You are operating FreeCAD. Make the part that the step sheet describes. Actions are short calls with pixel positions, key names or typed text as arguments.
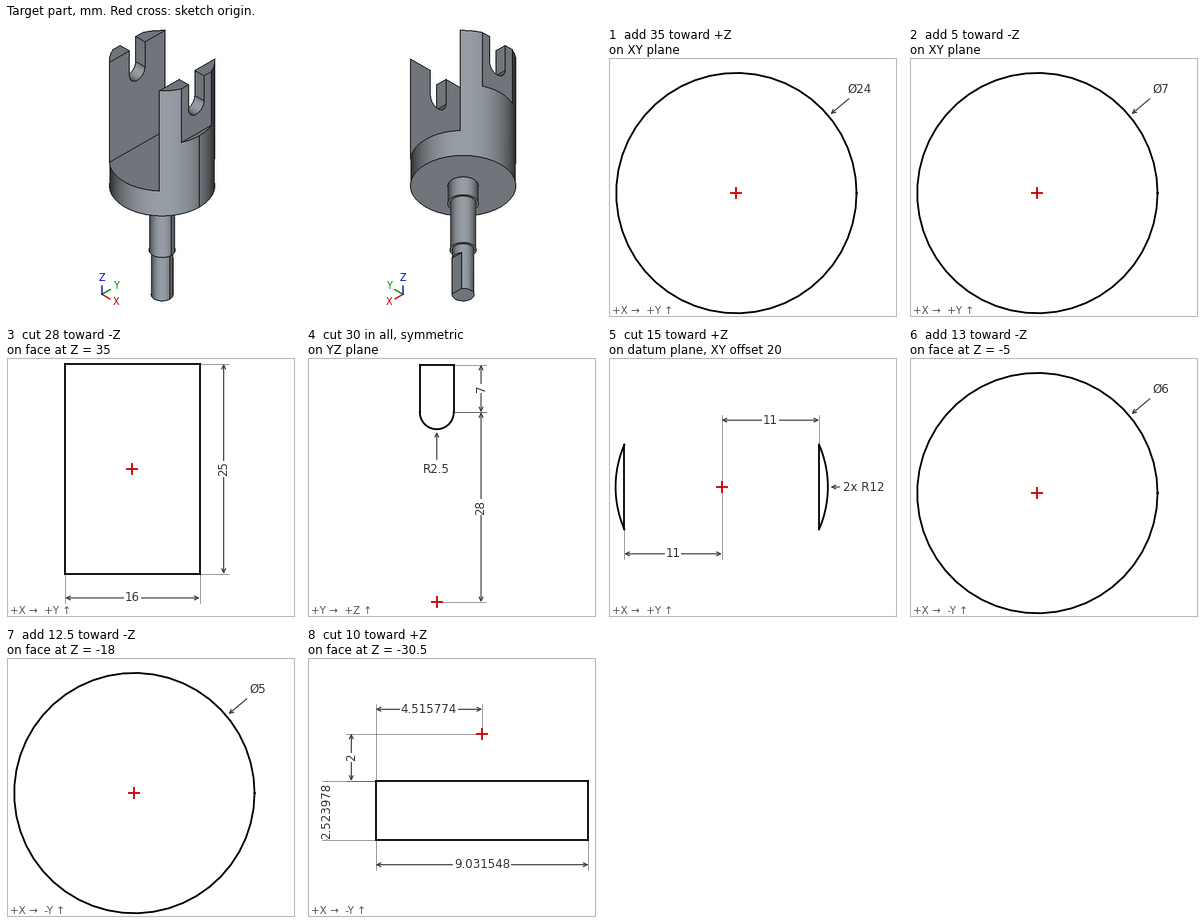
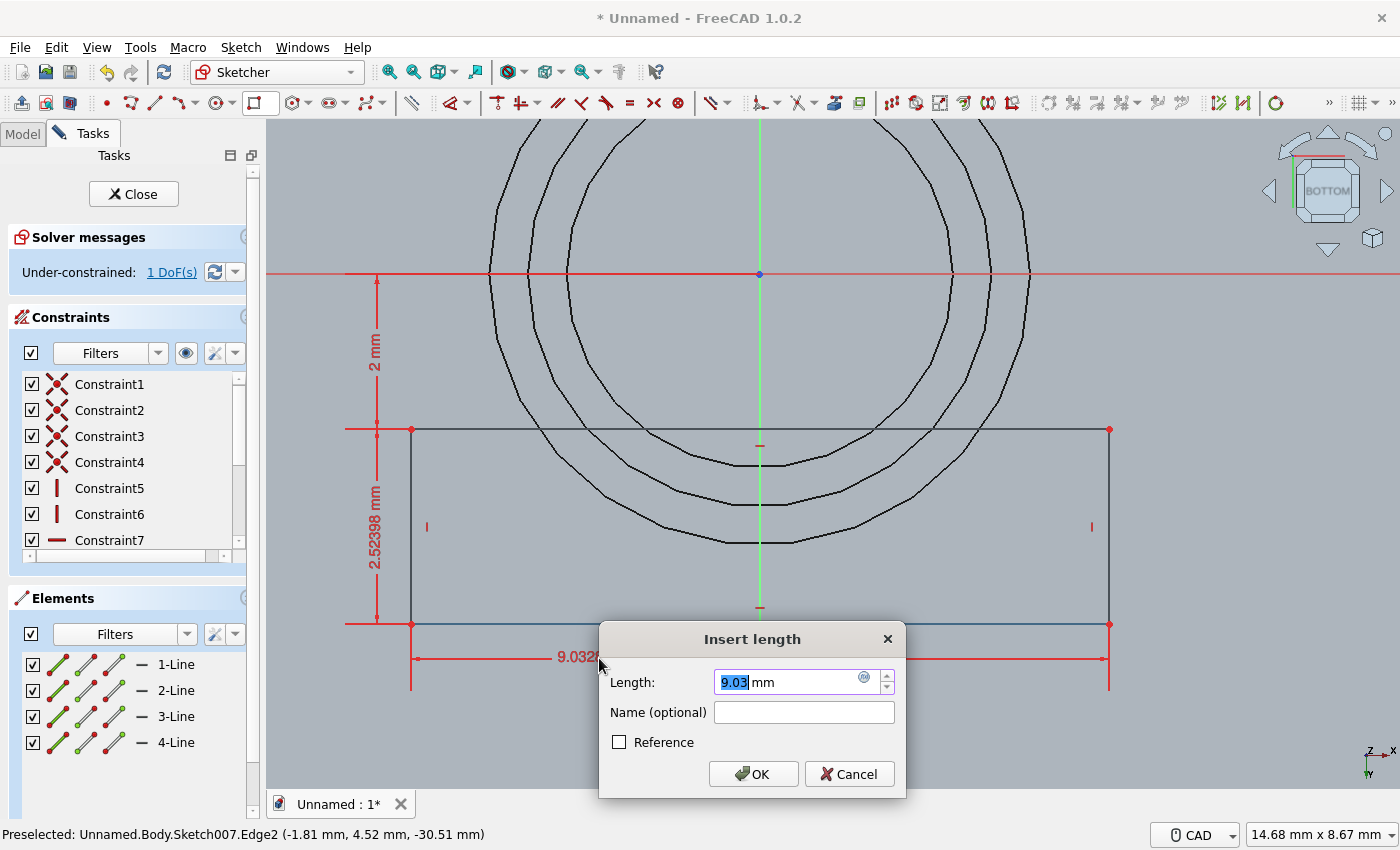
text(9.031548)
key(Return)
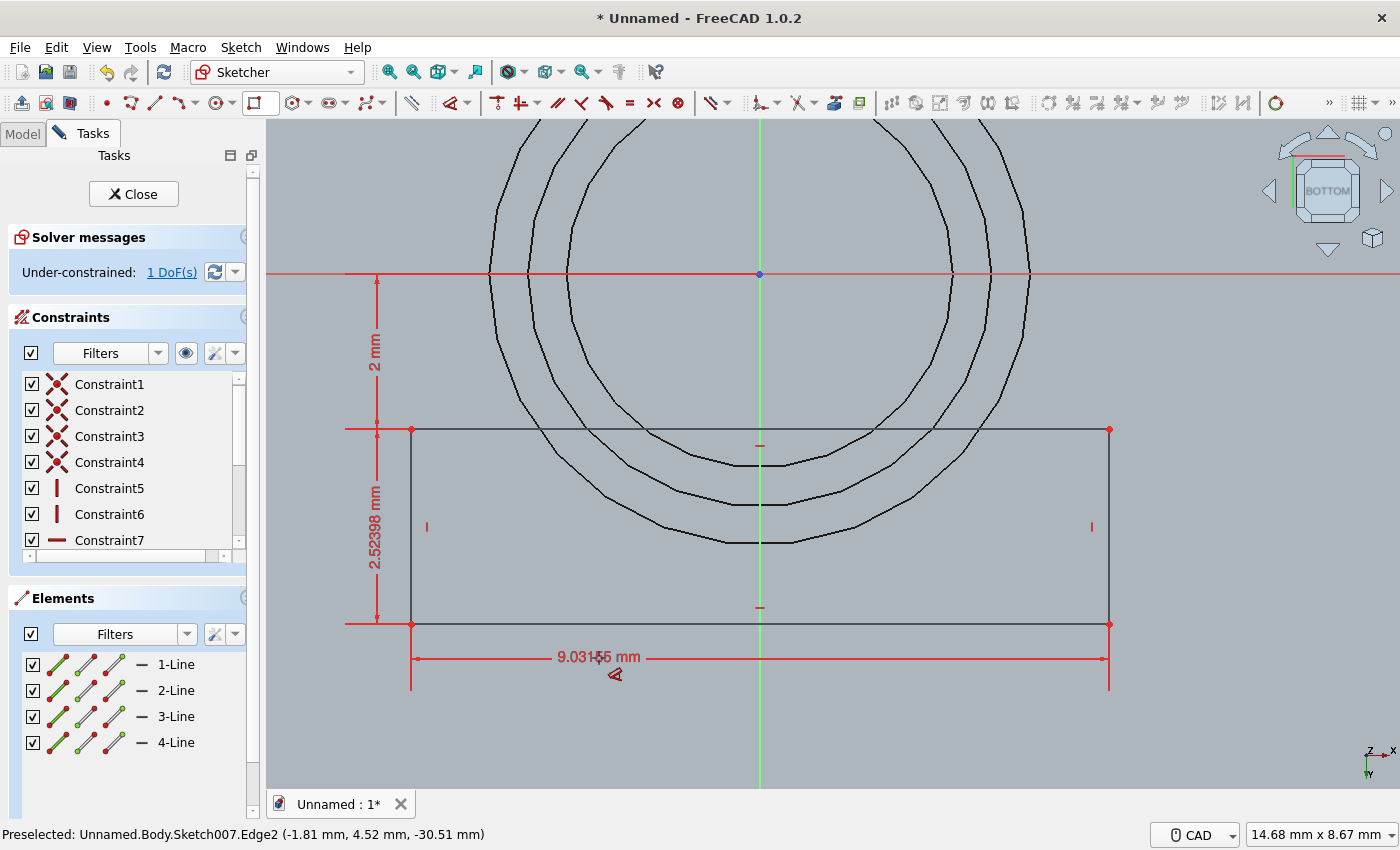
click(411, 429)
click(585, 240)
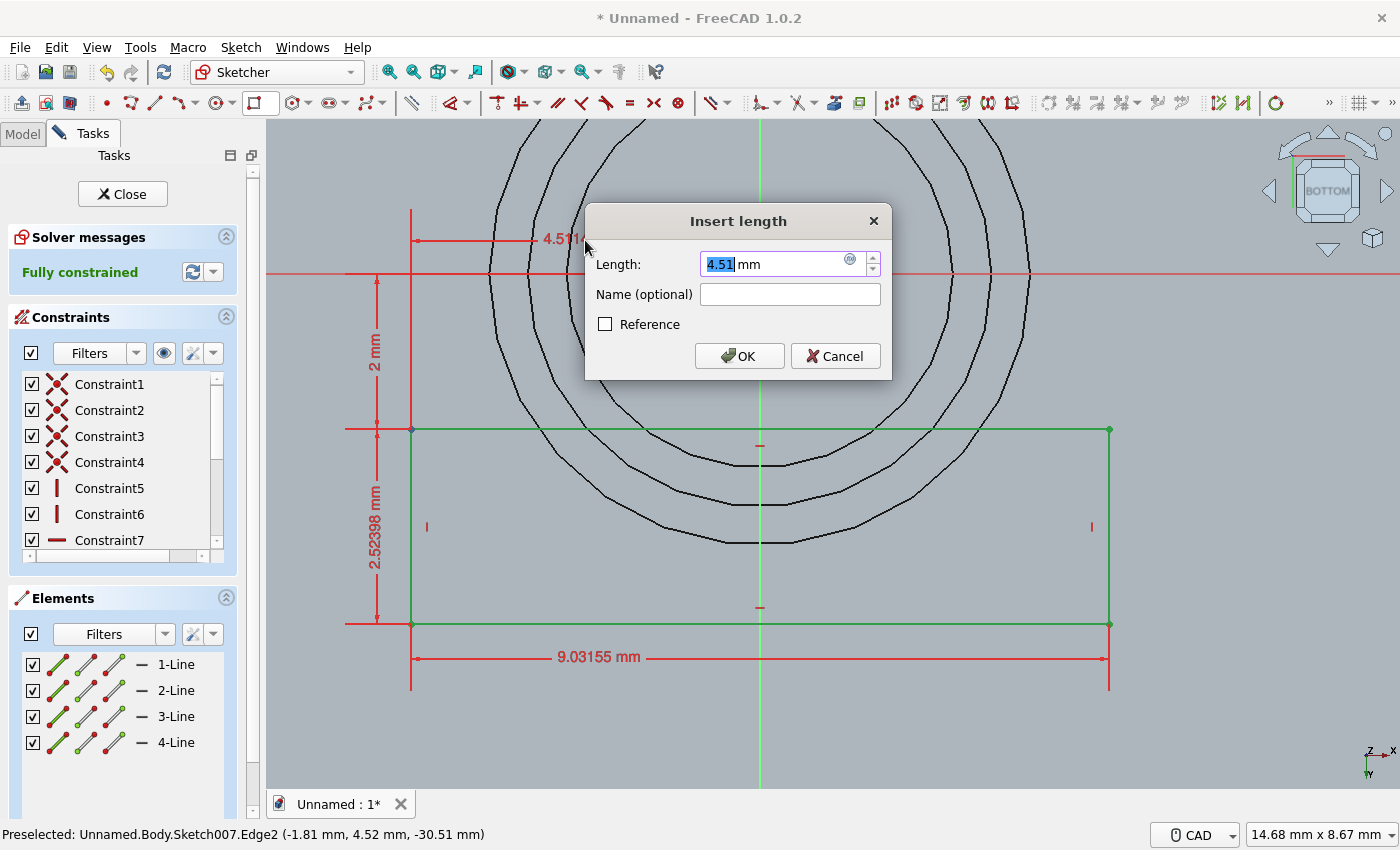
text(4.515774)
key(Return)
key(Escape)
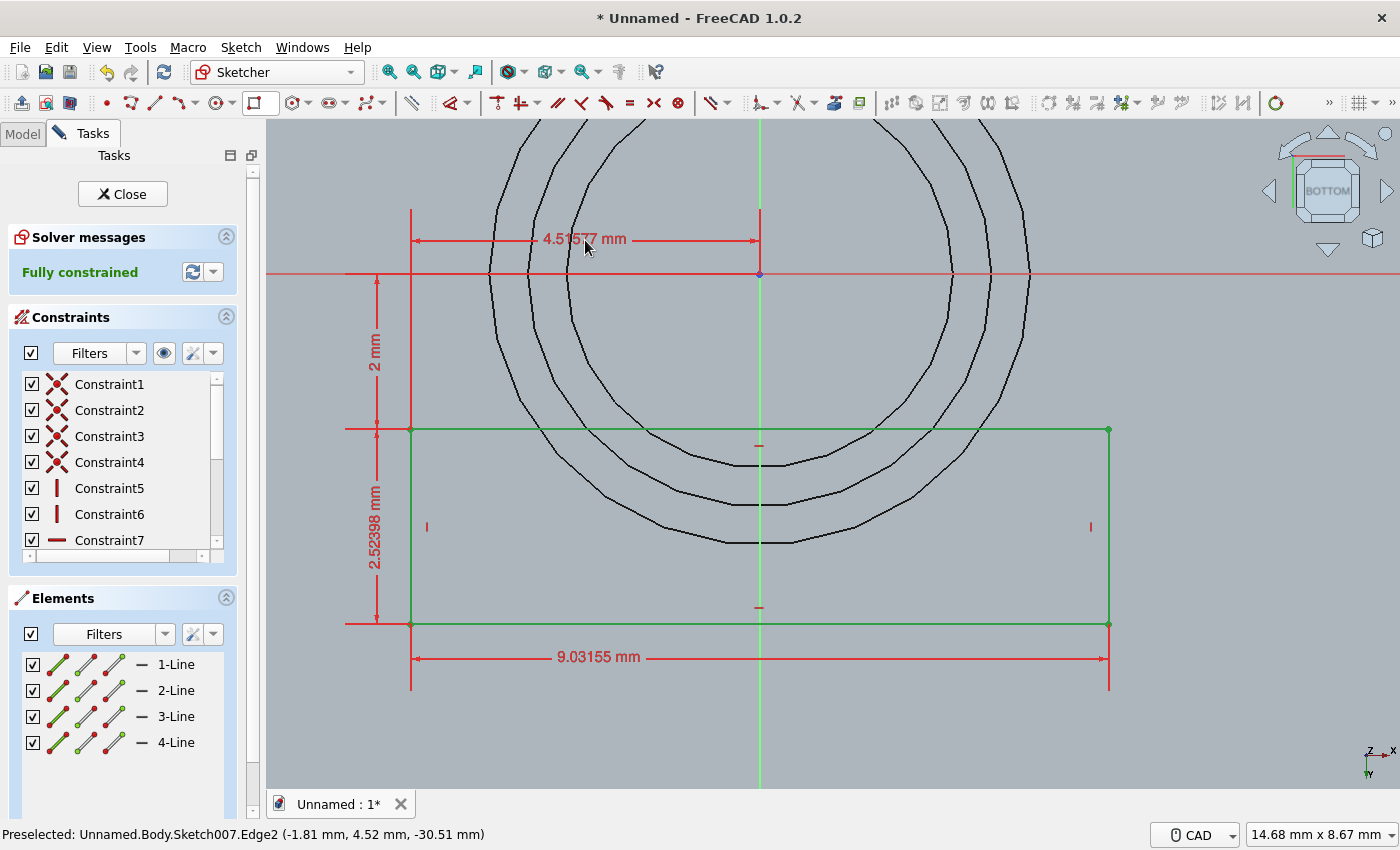
click(123, 194)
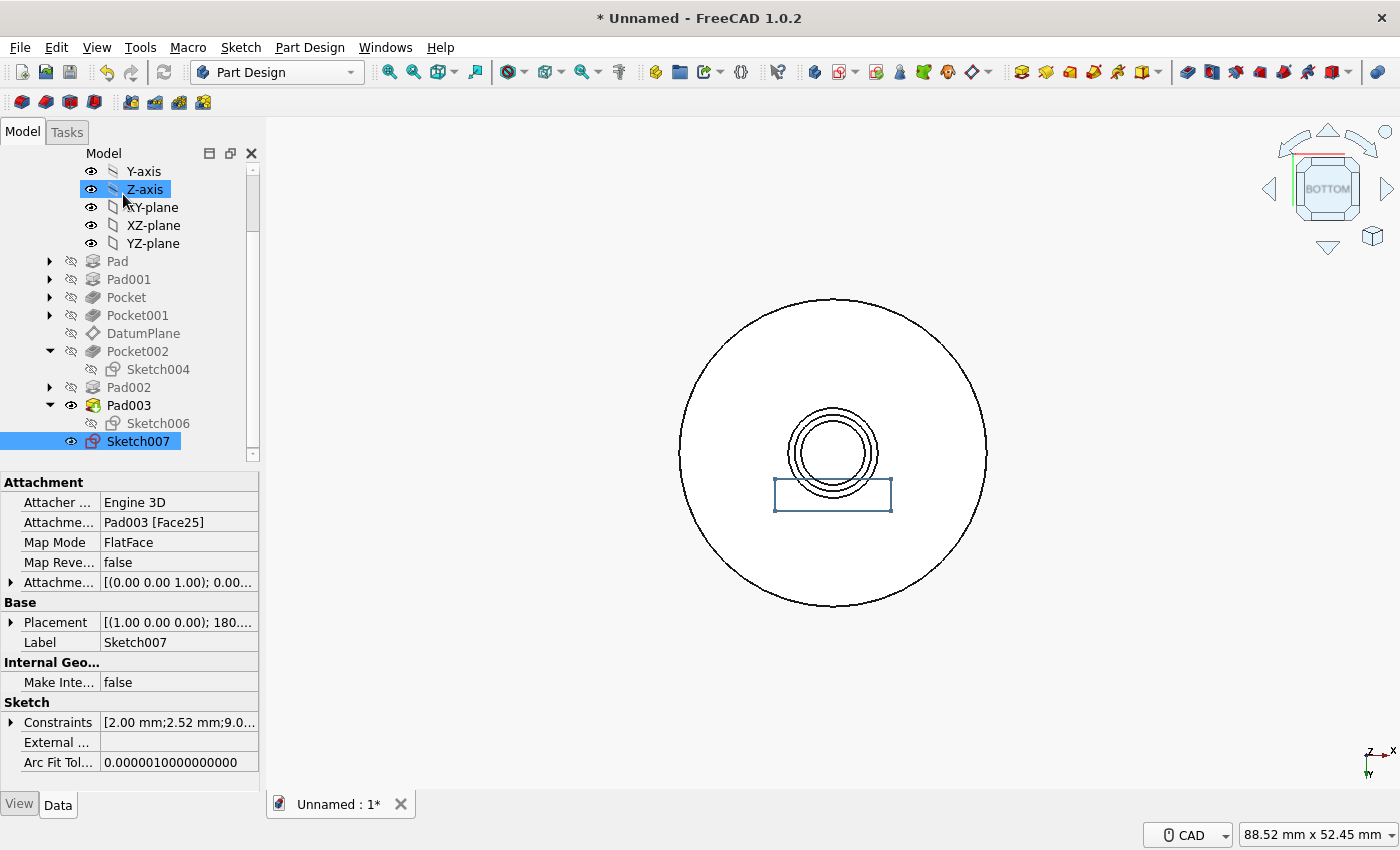
click(1188, 72)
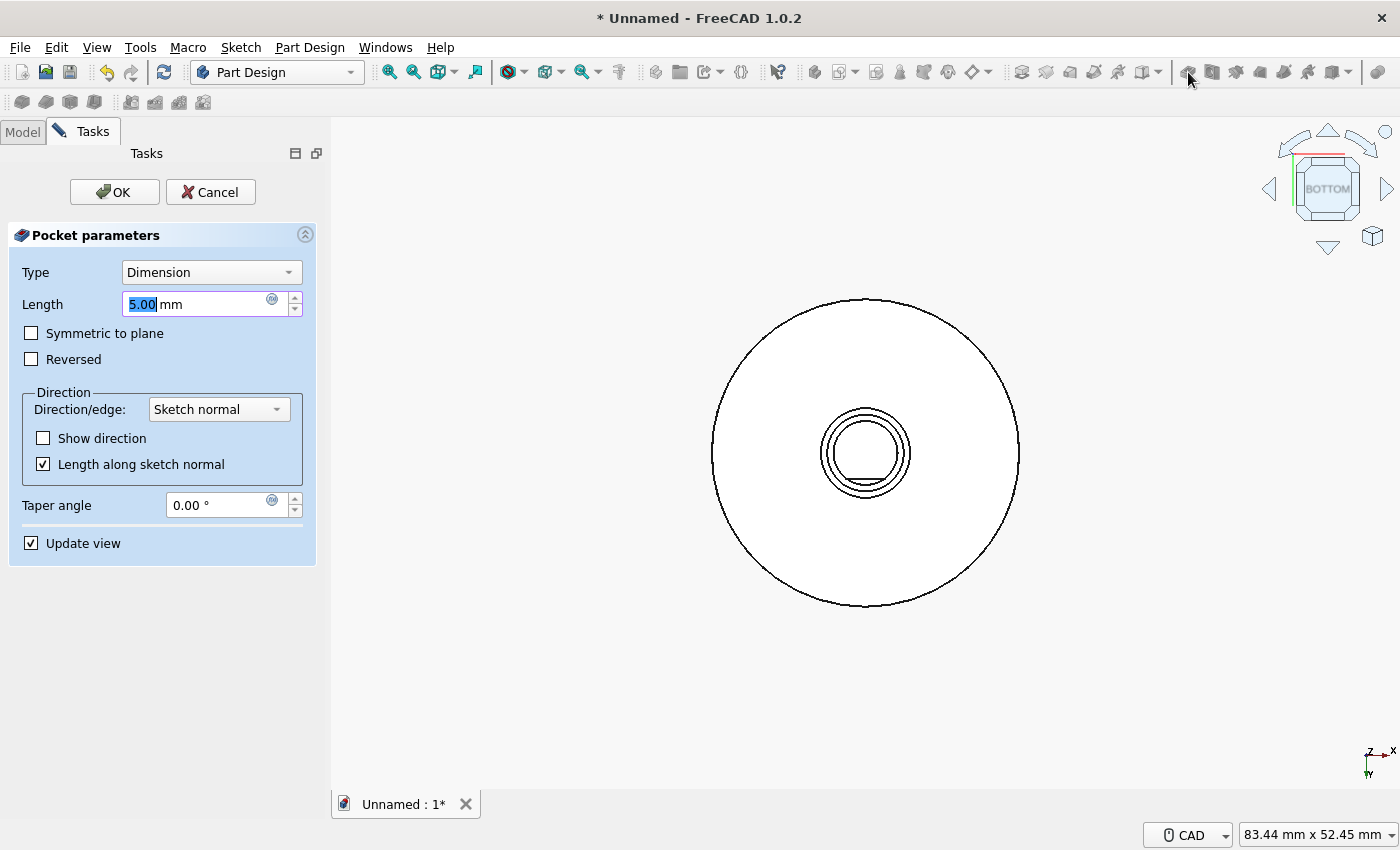
text(10)
key(Tab)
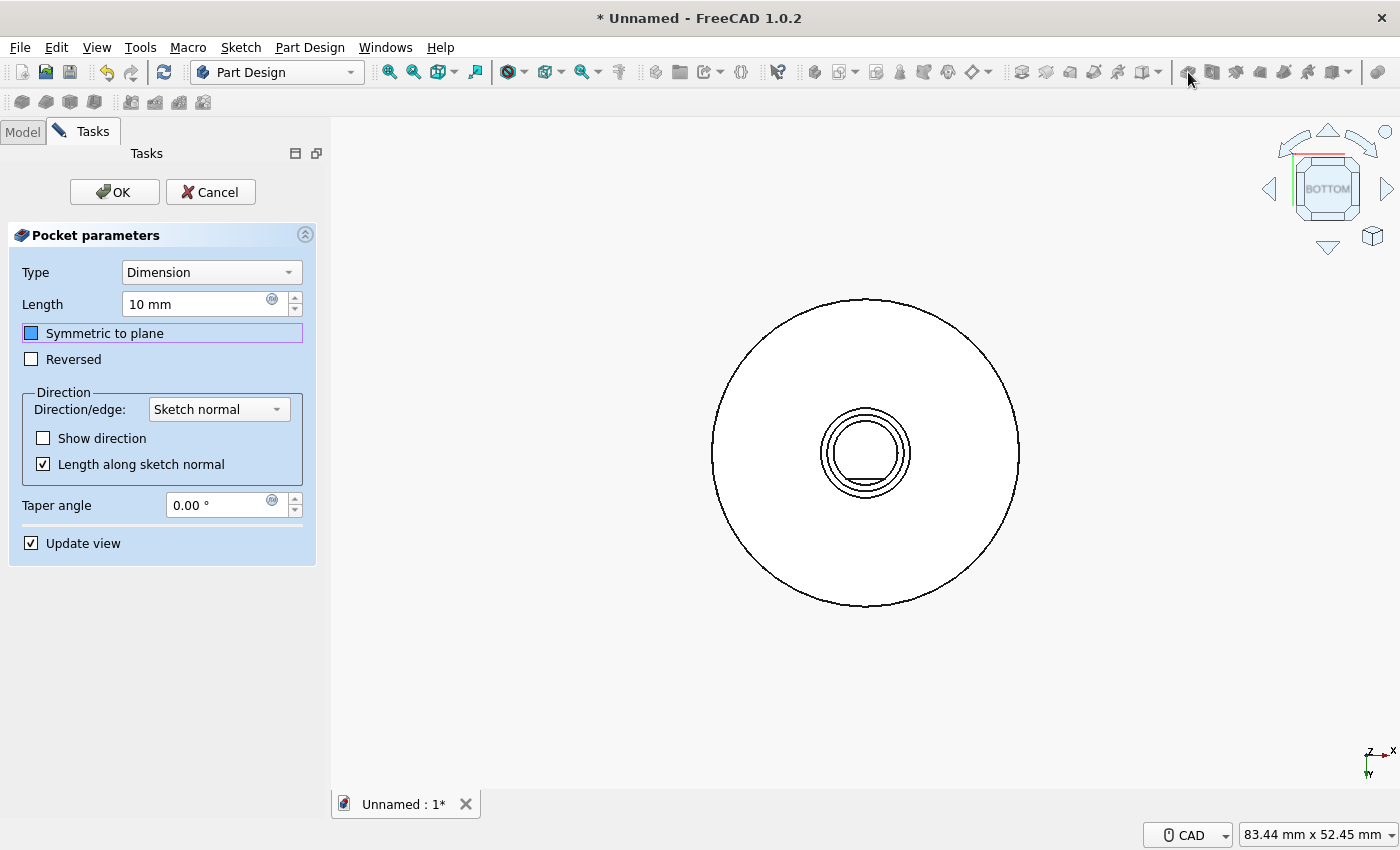
click(115, 192)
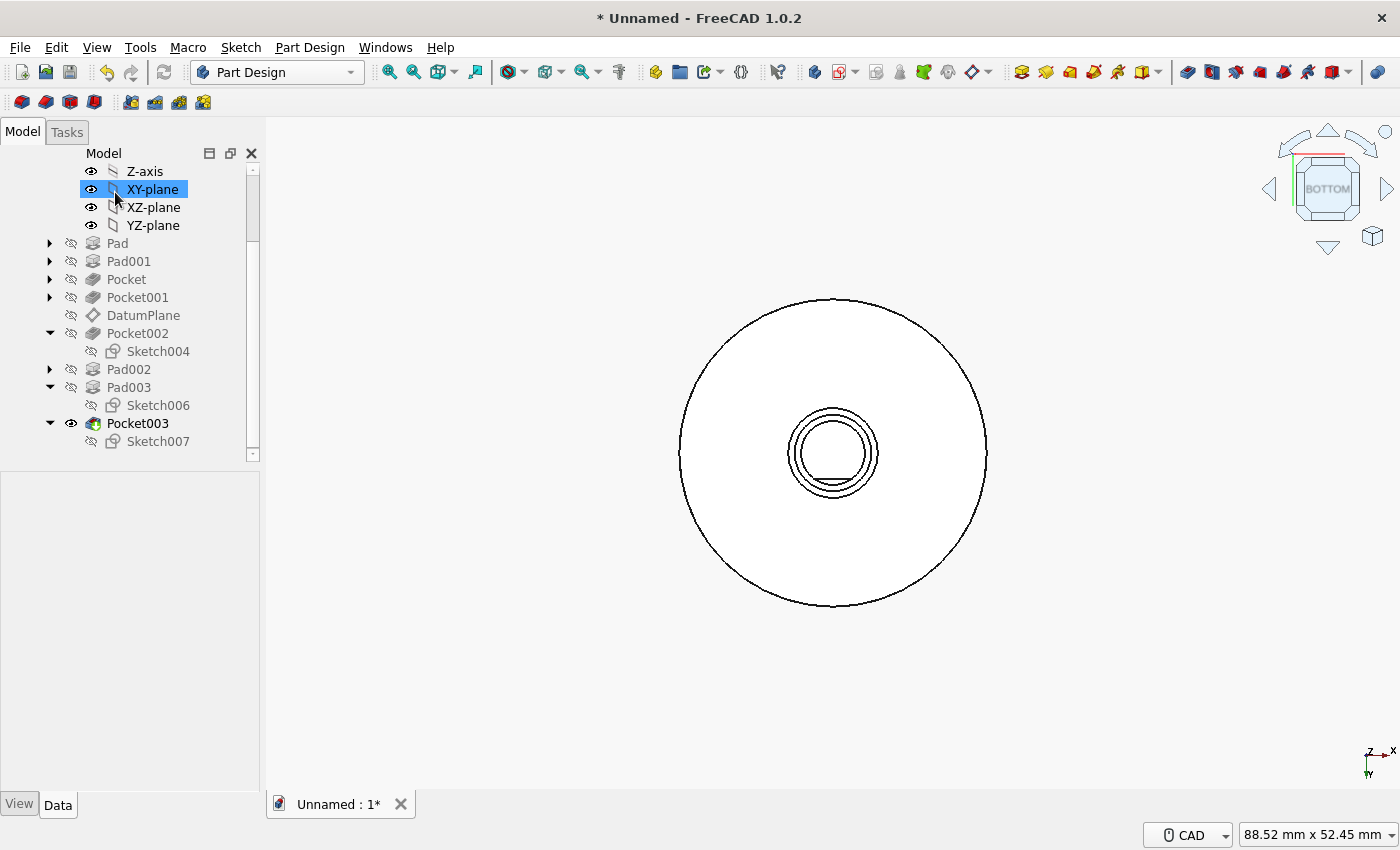
key(0)